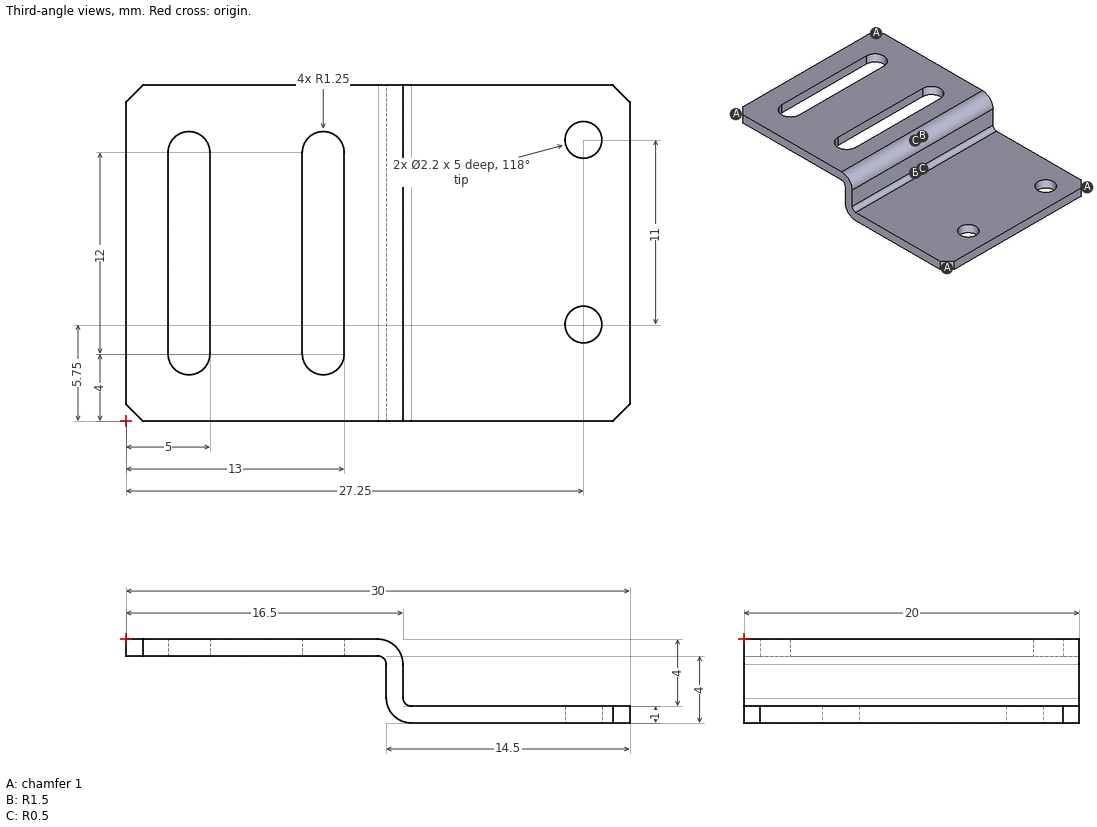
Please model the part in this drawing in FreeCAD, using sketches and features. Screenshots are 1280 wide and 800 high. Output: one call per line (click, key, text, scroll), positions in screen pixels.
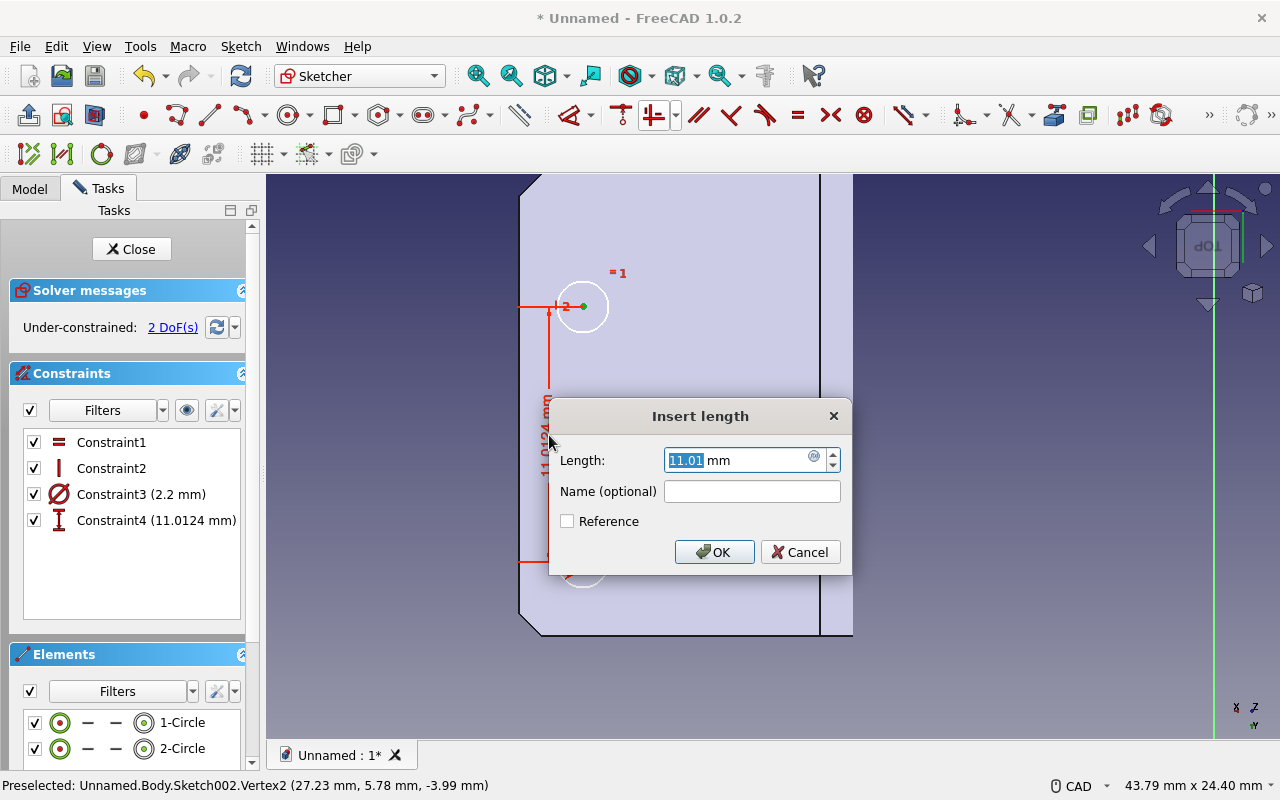
text(11)
key(Return)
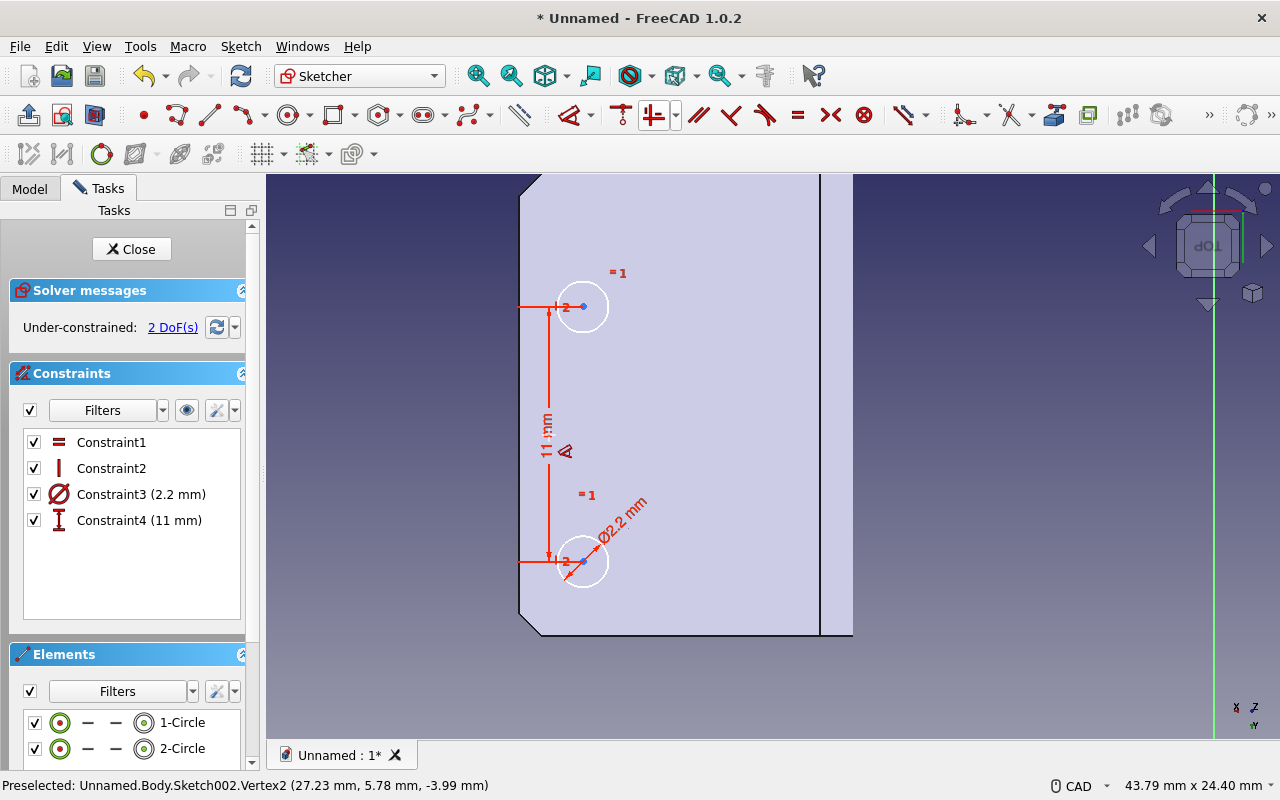
click(583, 307)
click(549, 255)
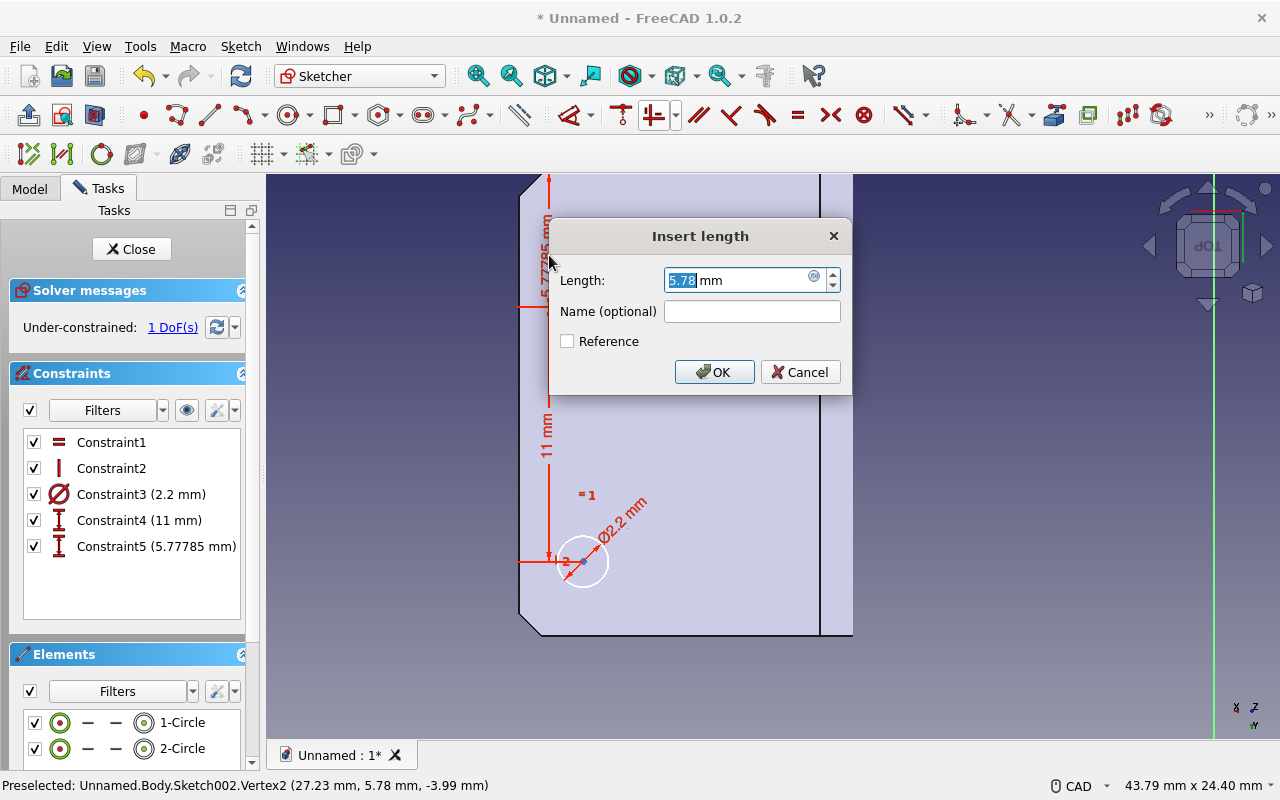
text(5.75)
key(Return)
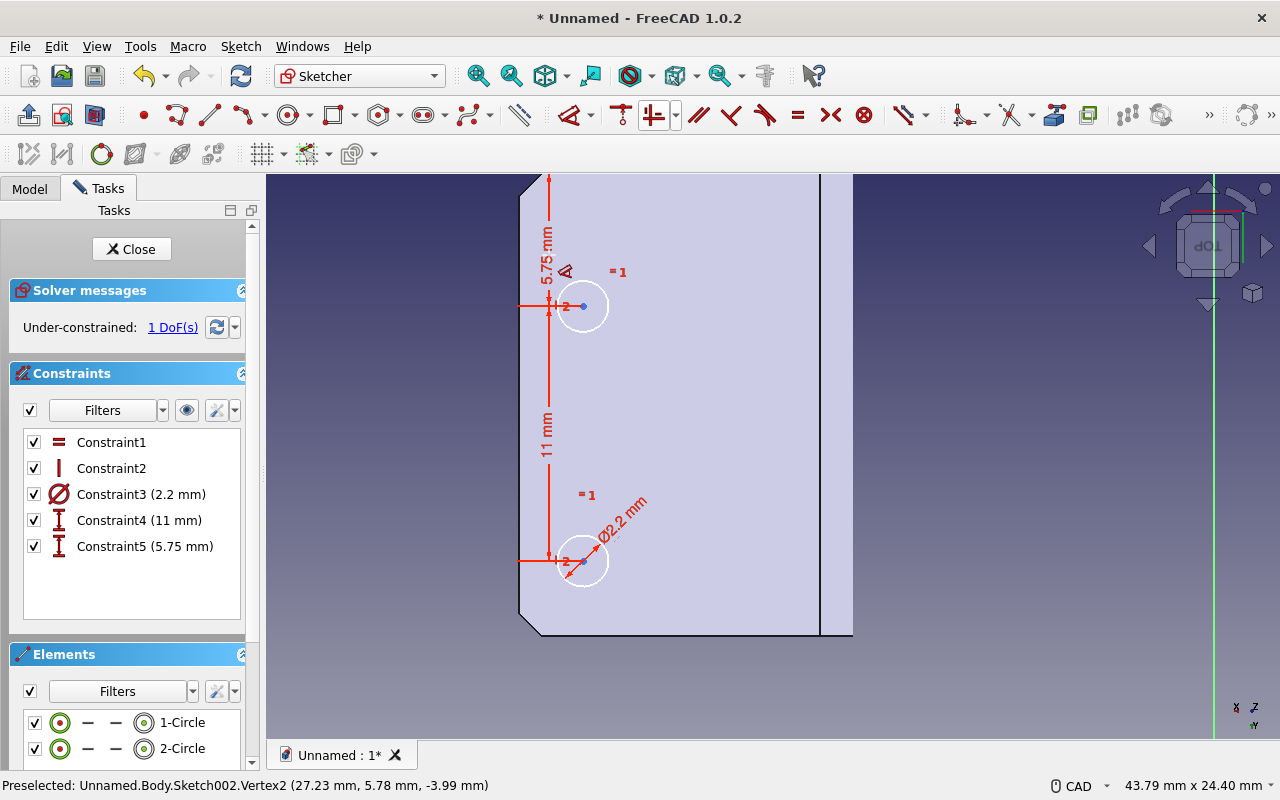
click(583, 561)
click(849, 595)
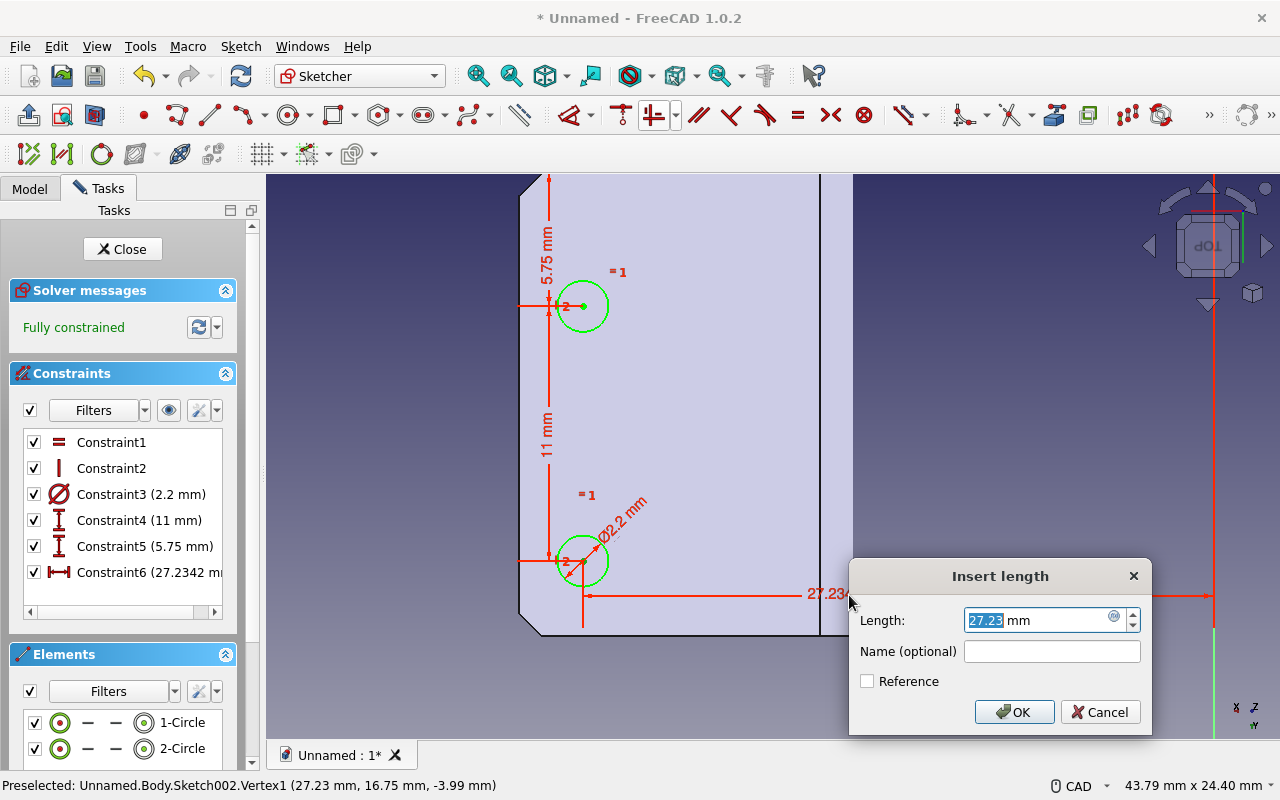
text(27.25)
key(Return)
key(Escape)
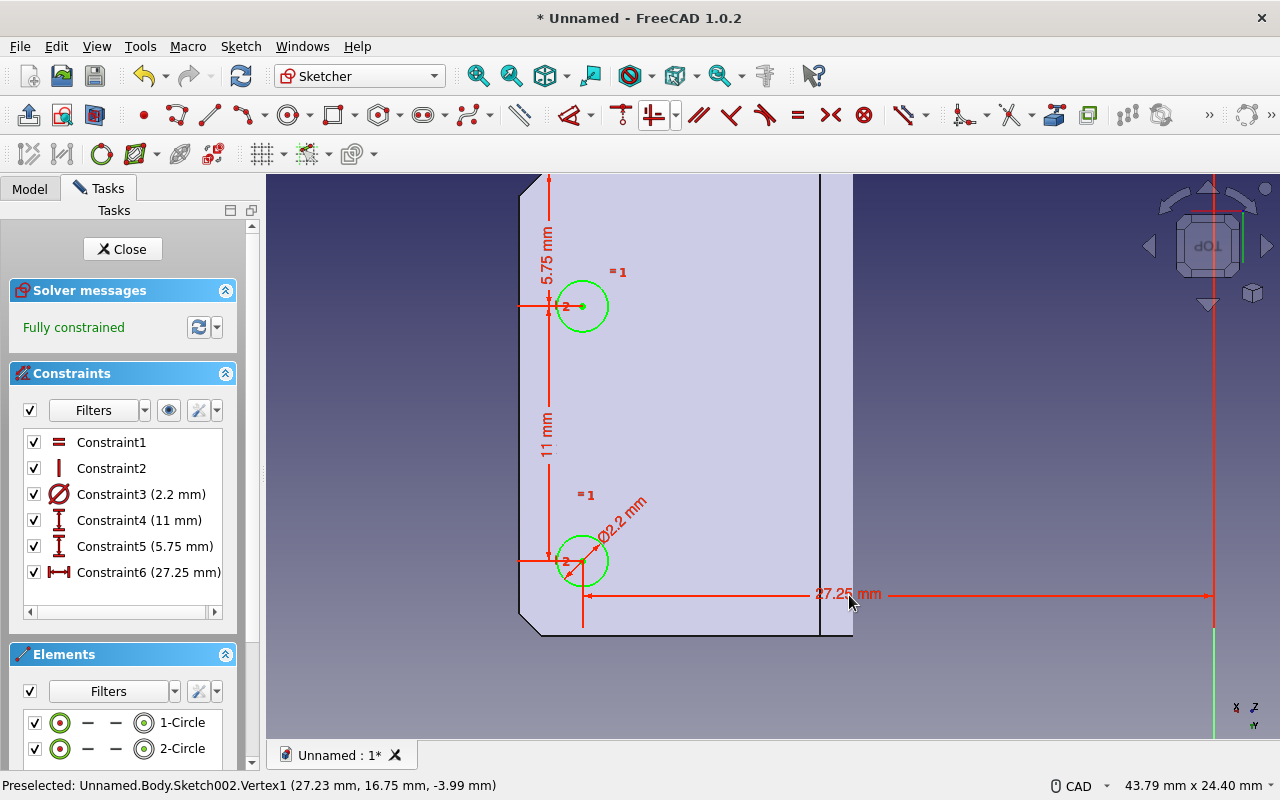
click(123, 249)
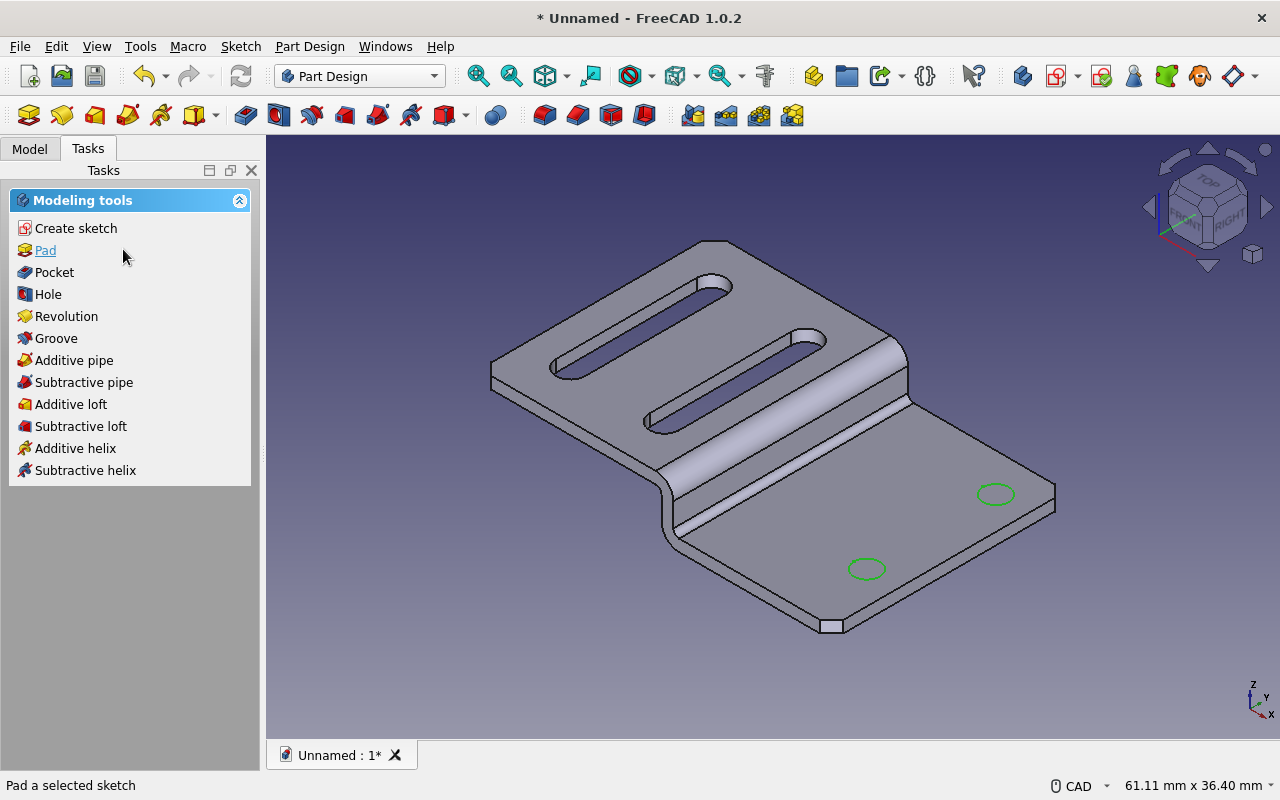
click(279, 116)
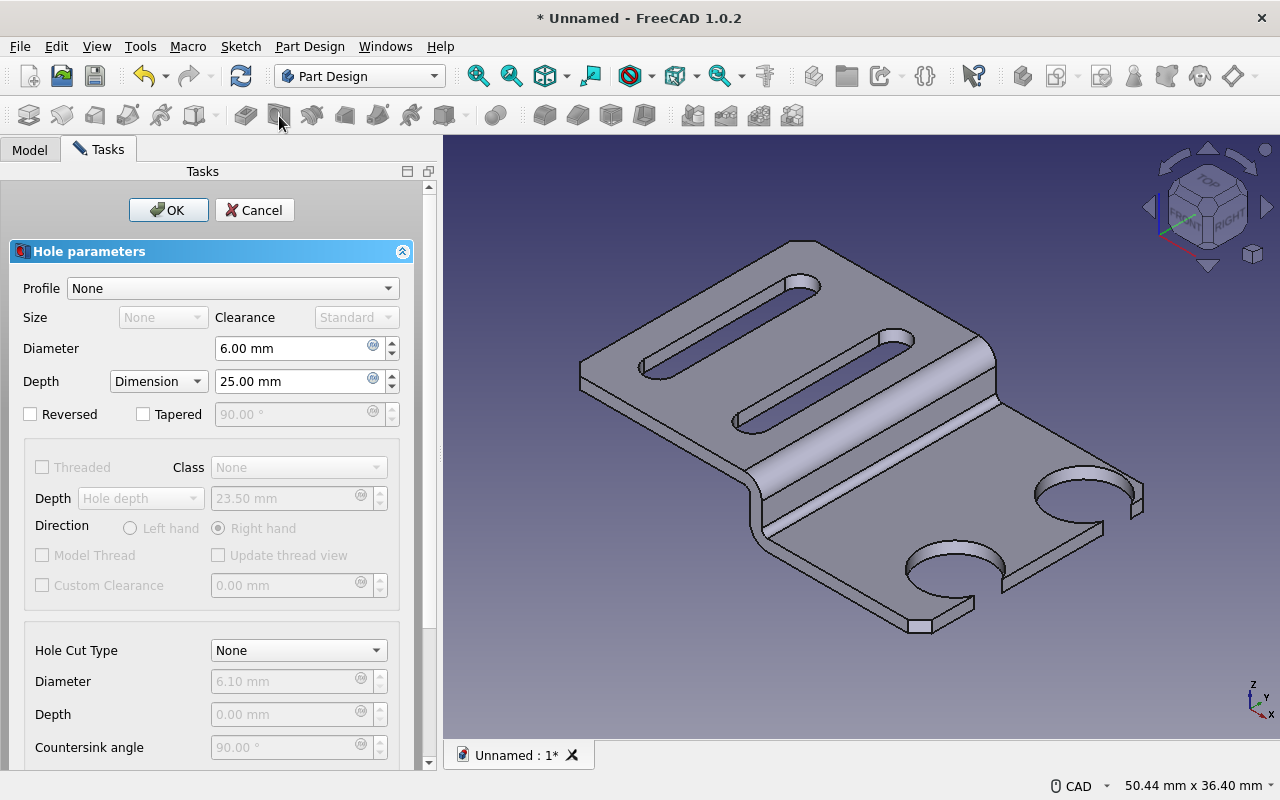
triple_click(300, 348)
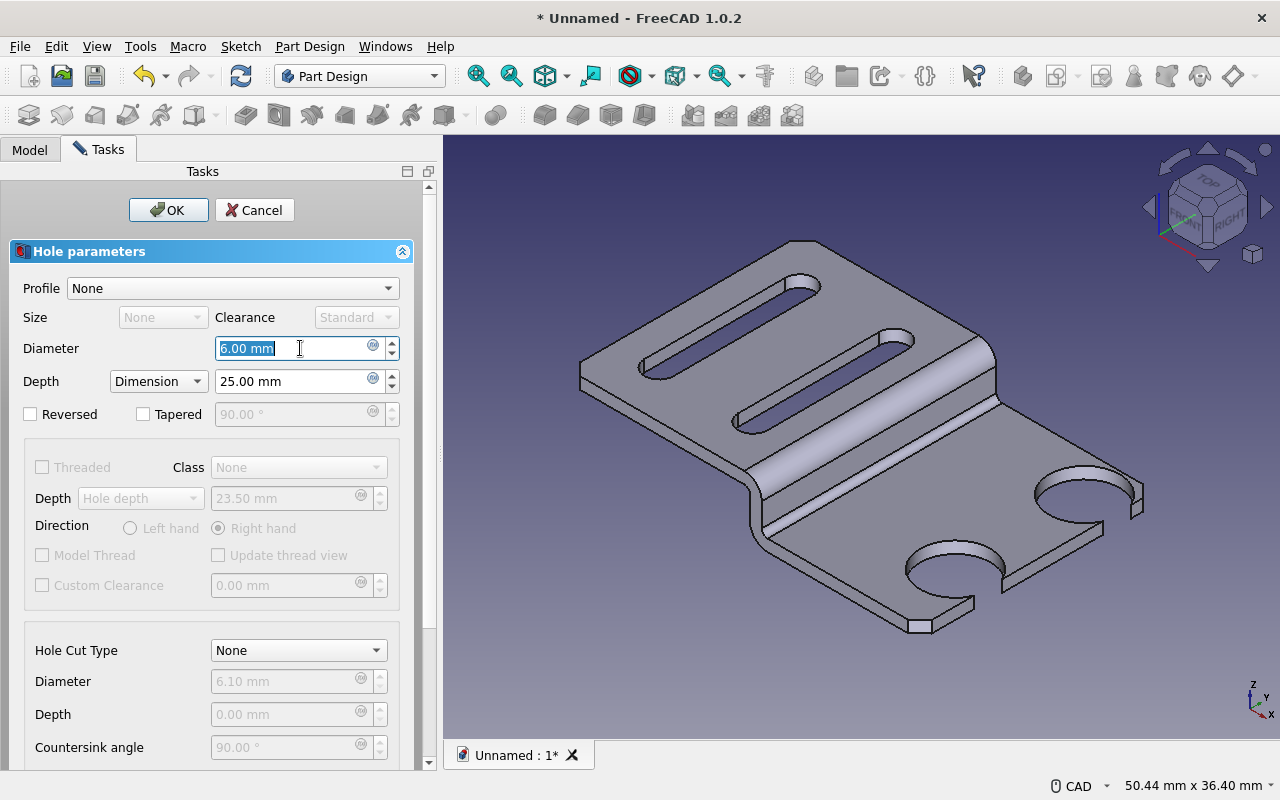
text(2.2)
key(Tab)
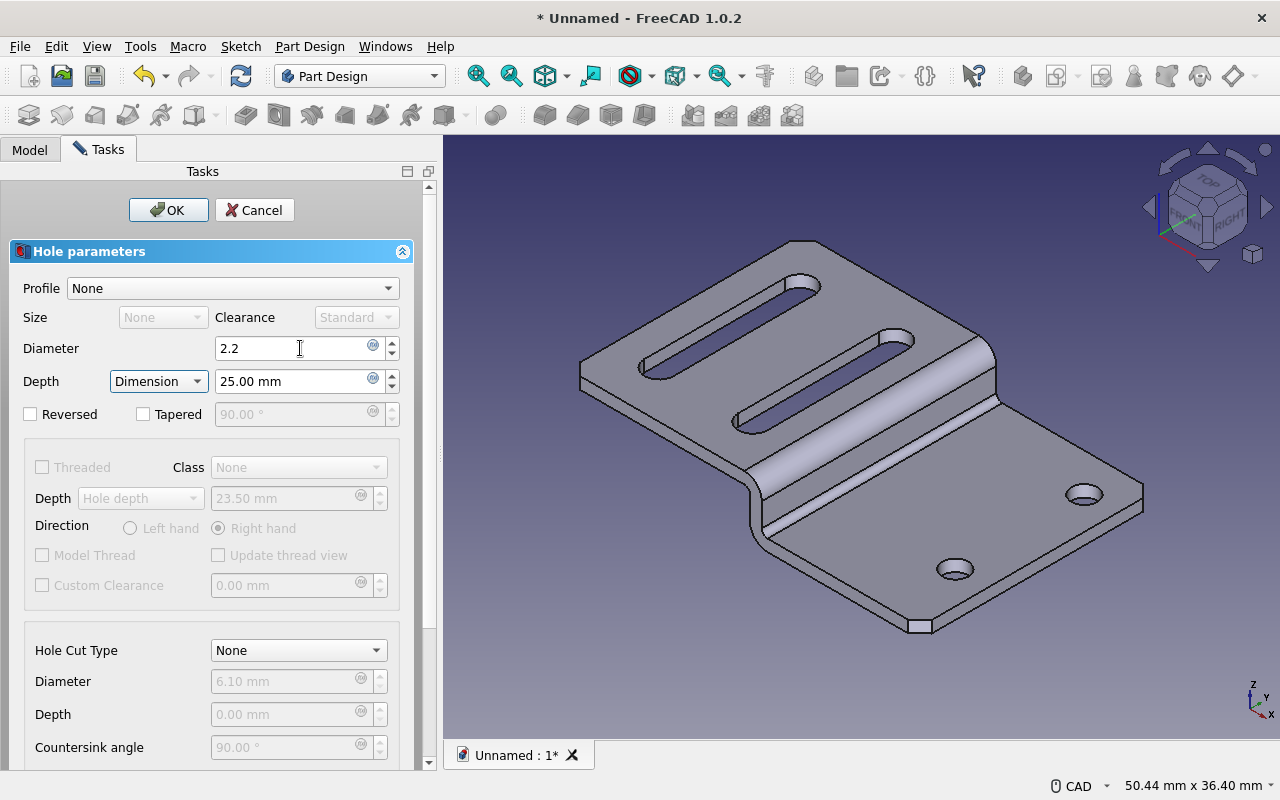
triple_click(300, 382)